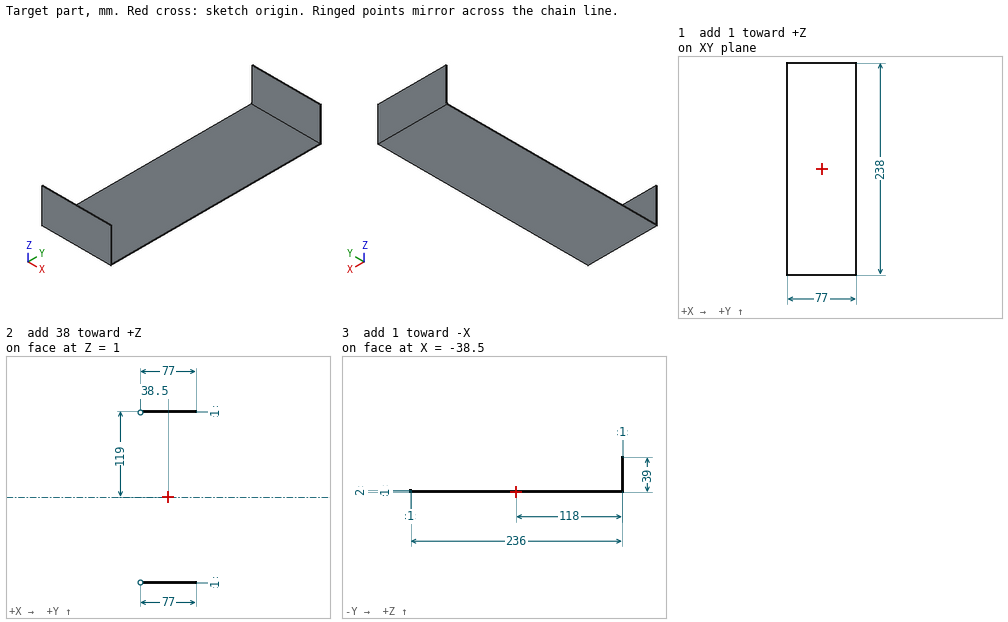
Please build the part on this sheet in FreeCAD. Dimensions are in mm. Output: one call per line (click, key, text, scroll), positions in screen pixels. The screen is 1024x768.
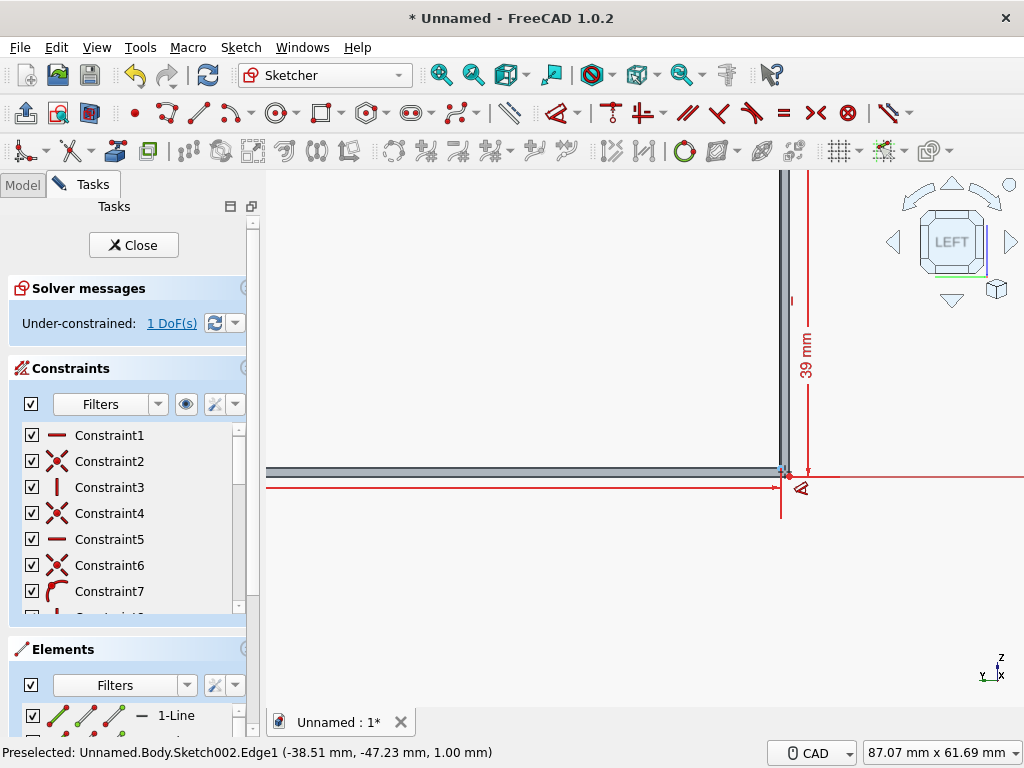
click(781, 468)
click(537, 511)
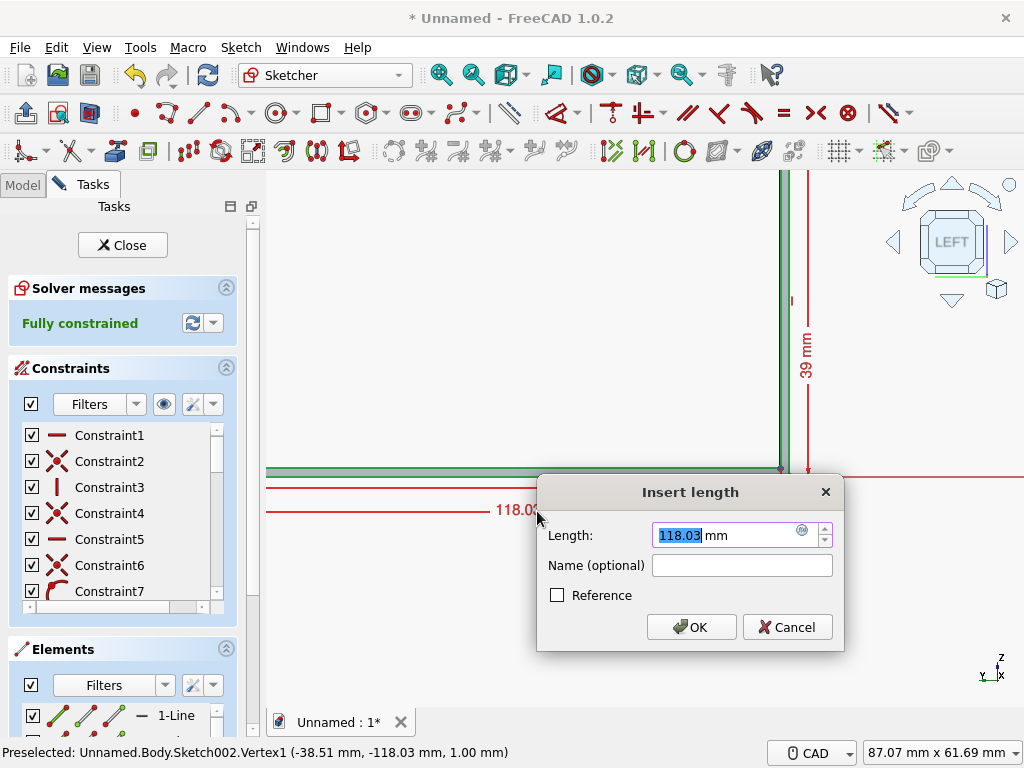
text(118)
key(Return)
key(Escape)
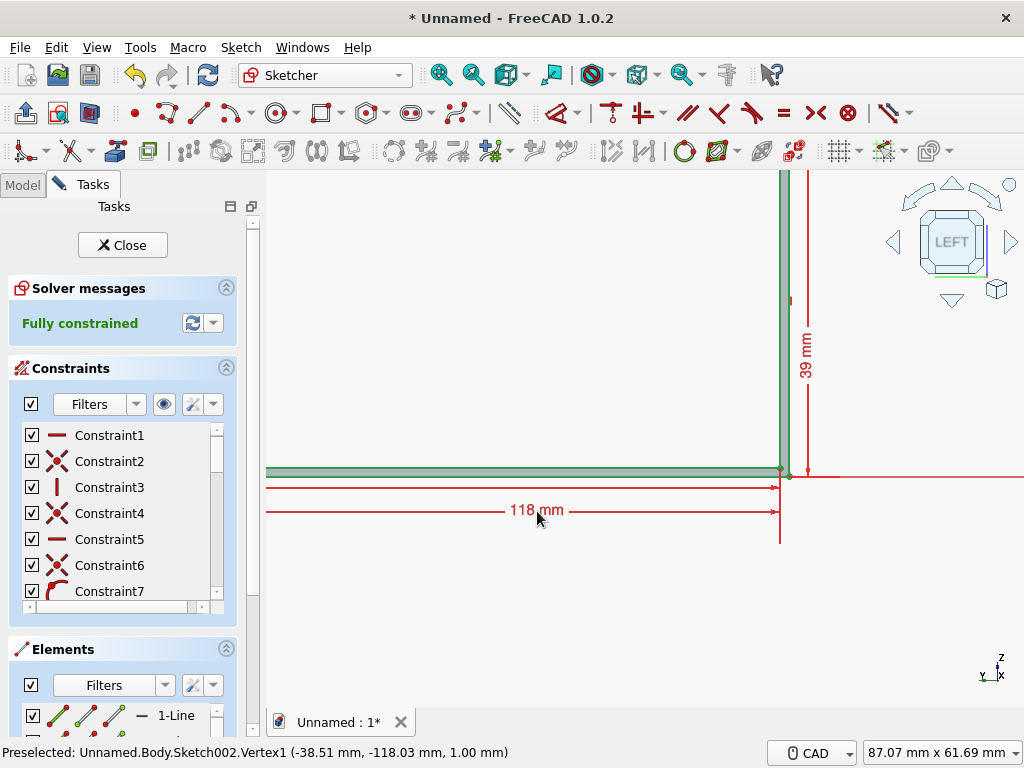
click(123, 245)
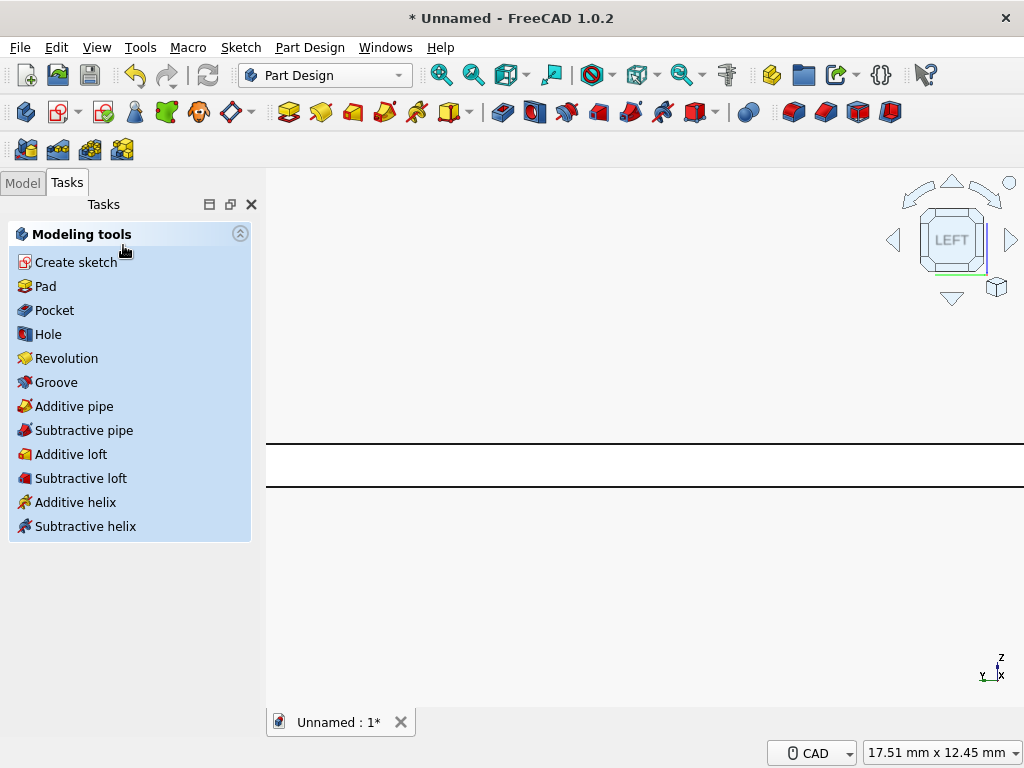
click(290, 112)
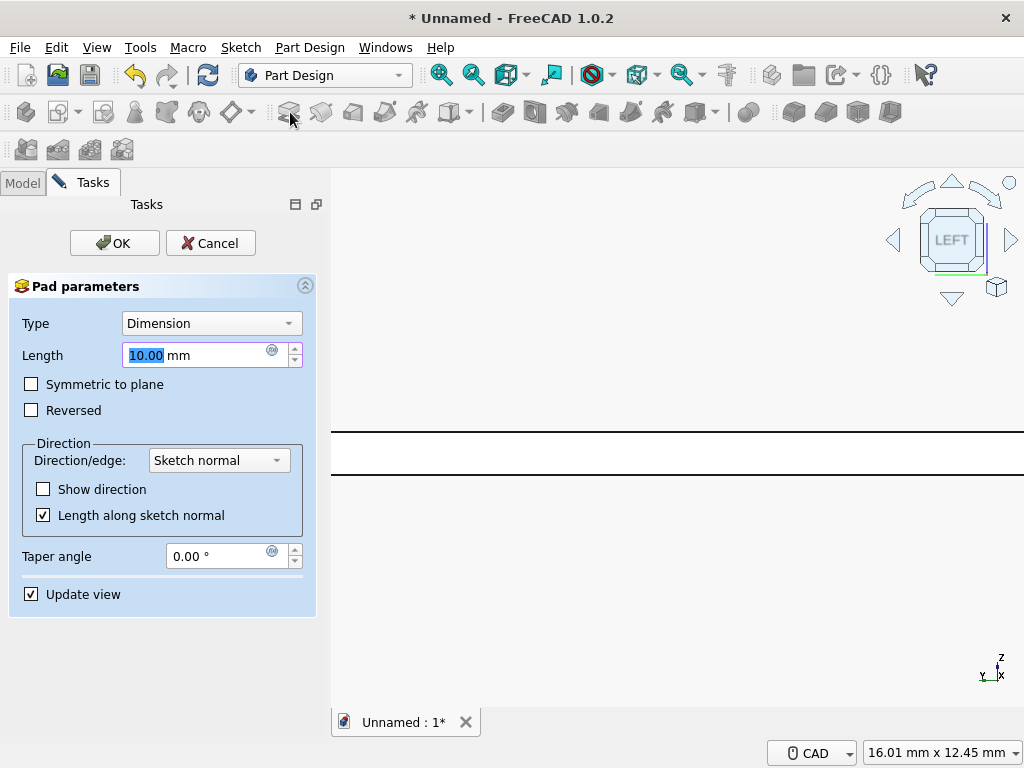
text(1)
key(Tab)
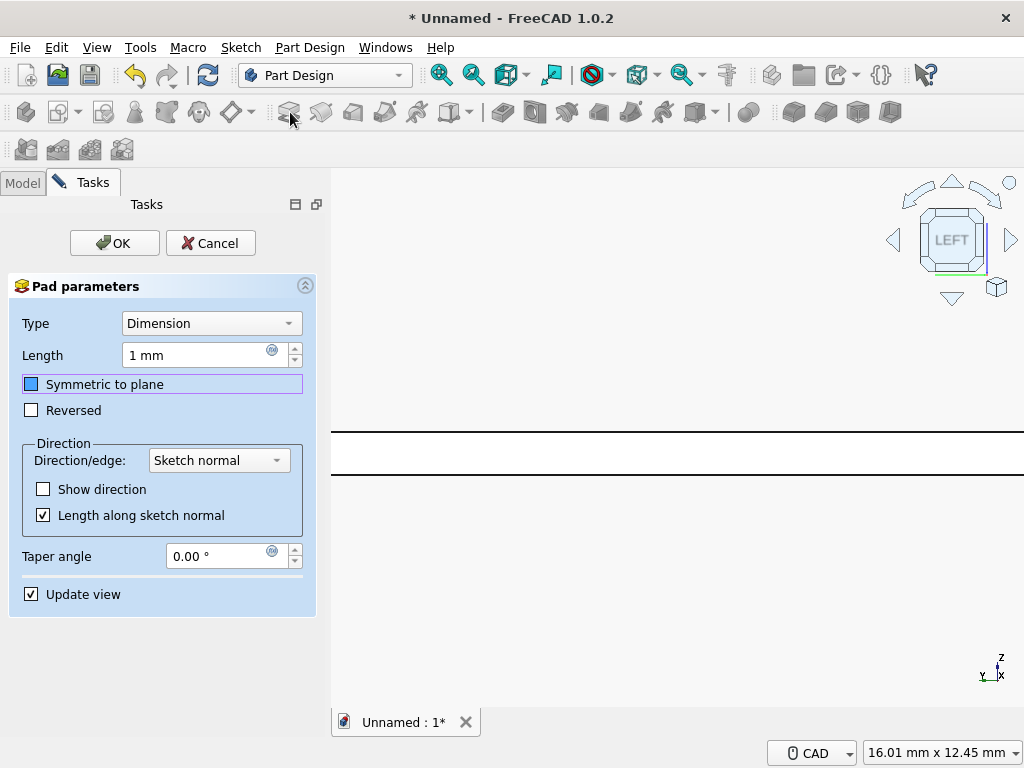
click(115, 243)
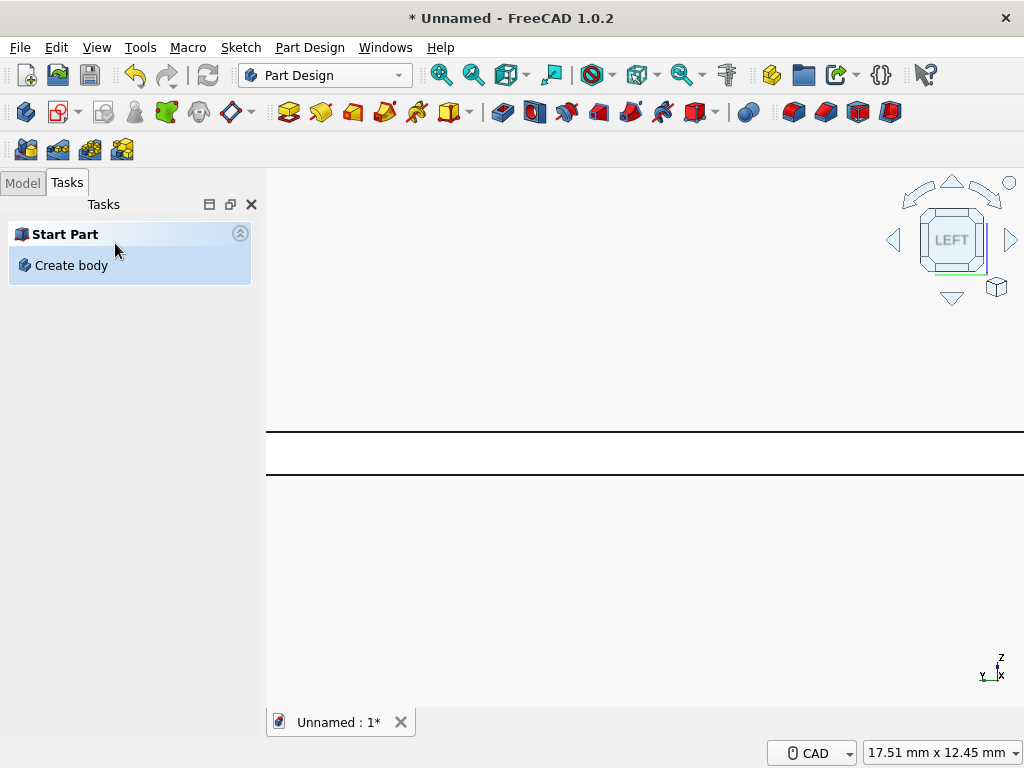
key(0)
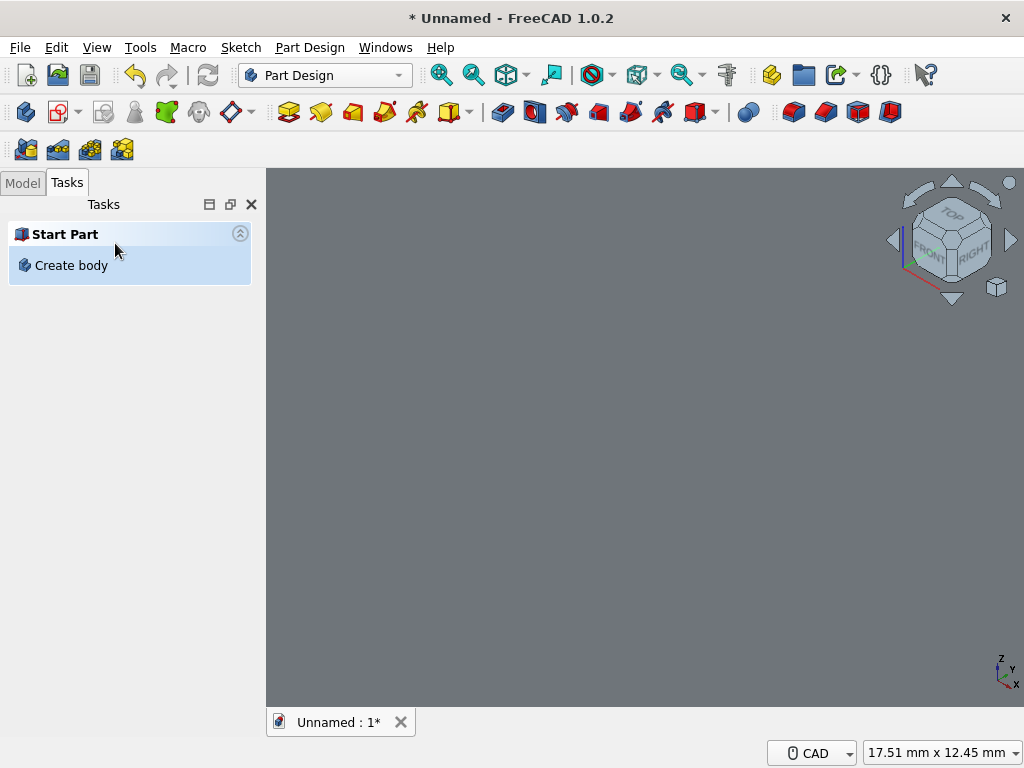
click(442, 76)